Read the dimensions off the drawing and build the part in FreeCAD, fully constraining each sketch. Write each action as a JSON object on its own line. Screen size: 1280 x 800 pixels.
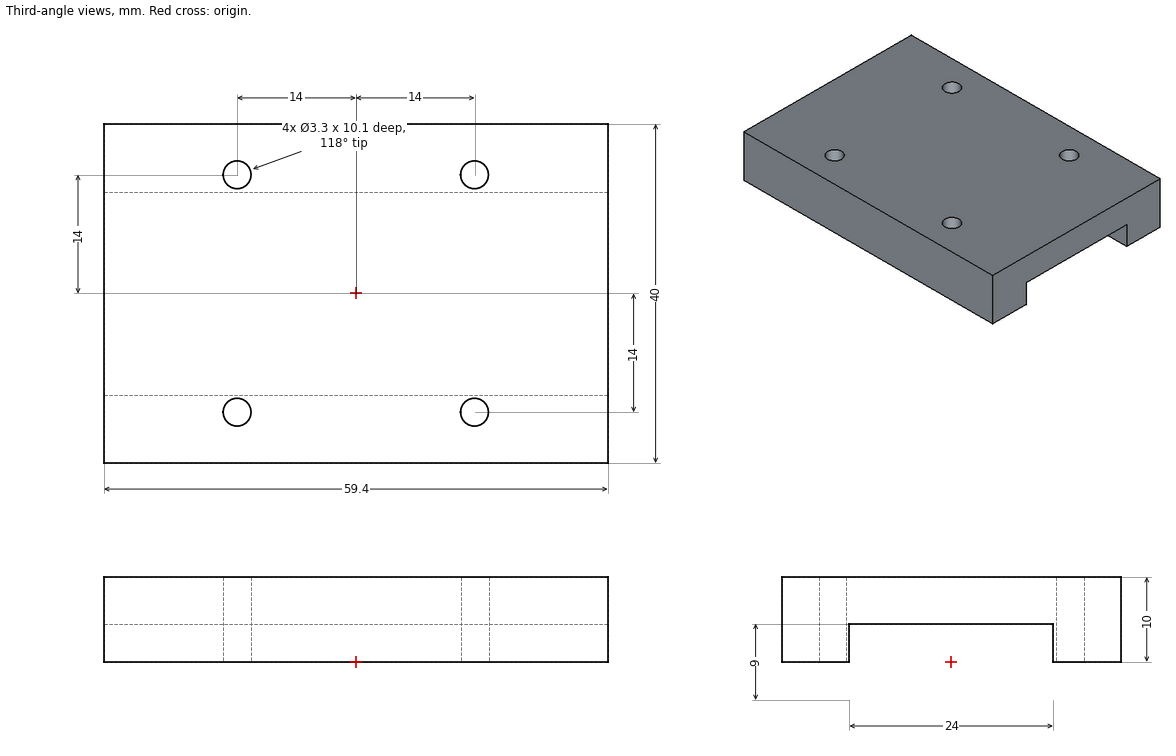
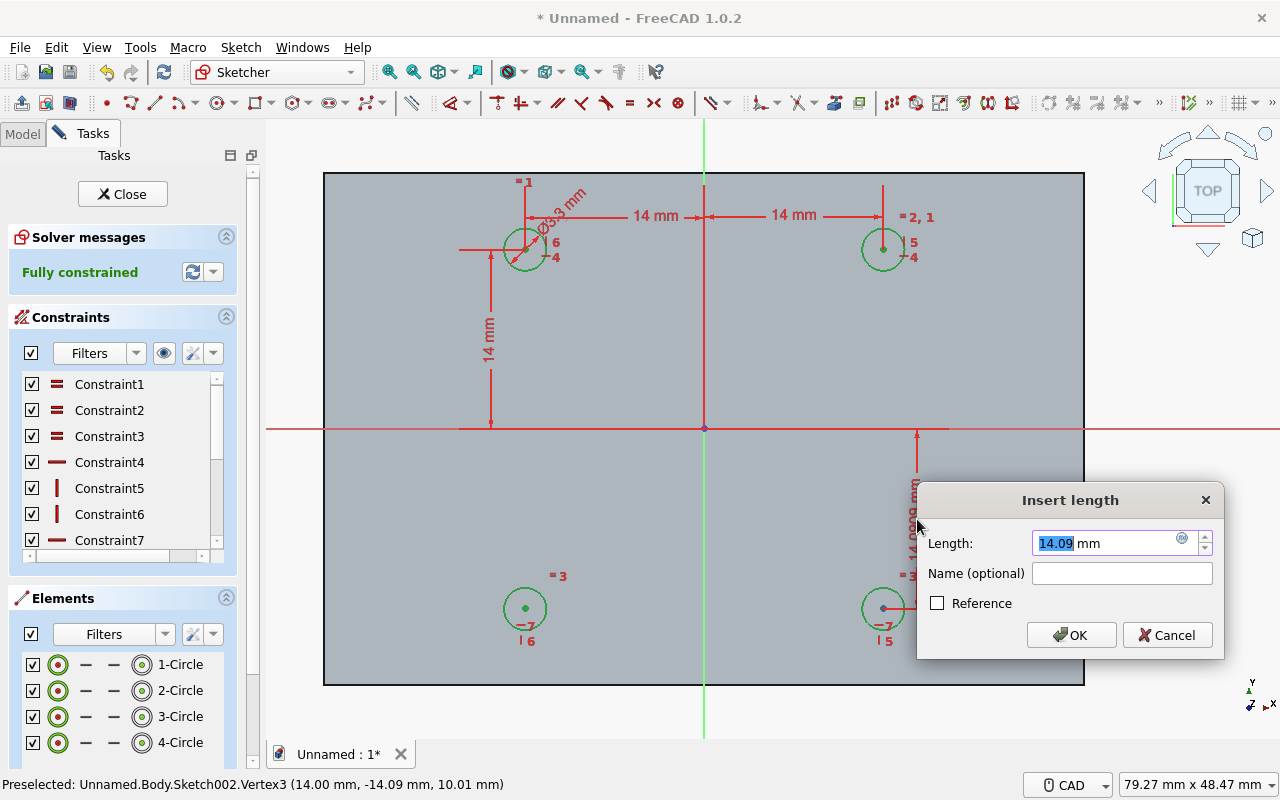
{"action": "type", "text": "14"}
{"action": "key", "text": "Return"}
{"action": "key", "text": "Escape"}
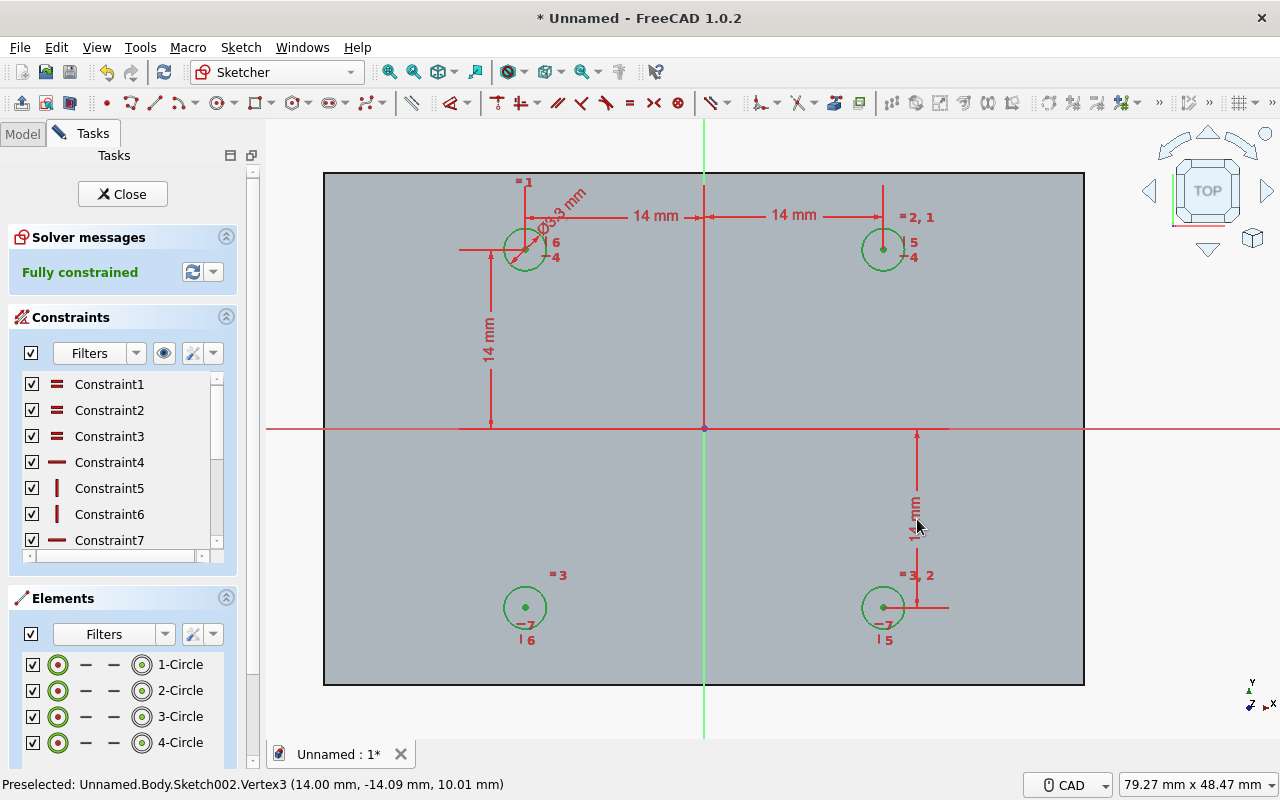
{"action": "left_click", "coordinate": [123, 194]}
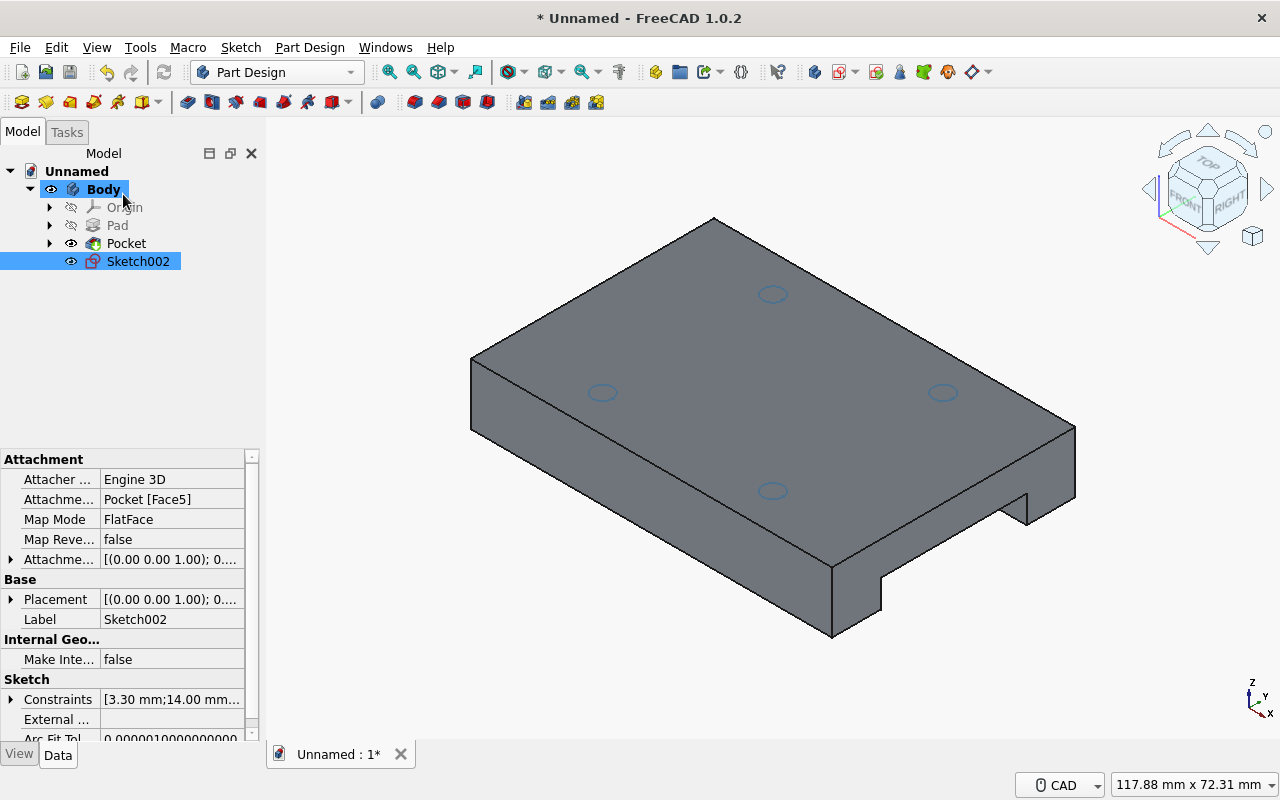
{"action": "left_click", "coordinate": [212, 102]}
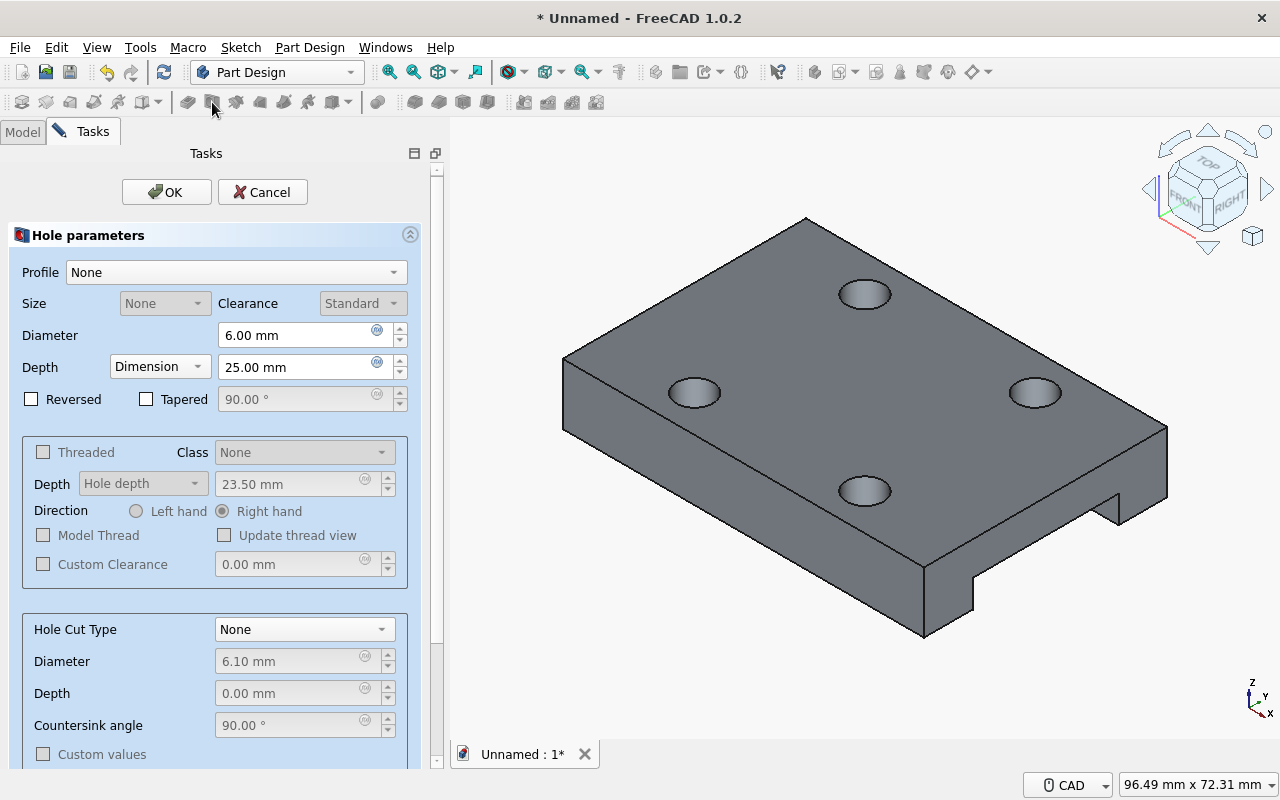
{"action": "triple_click", "coordinate": [305, 335]}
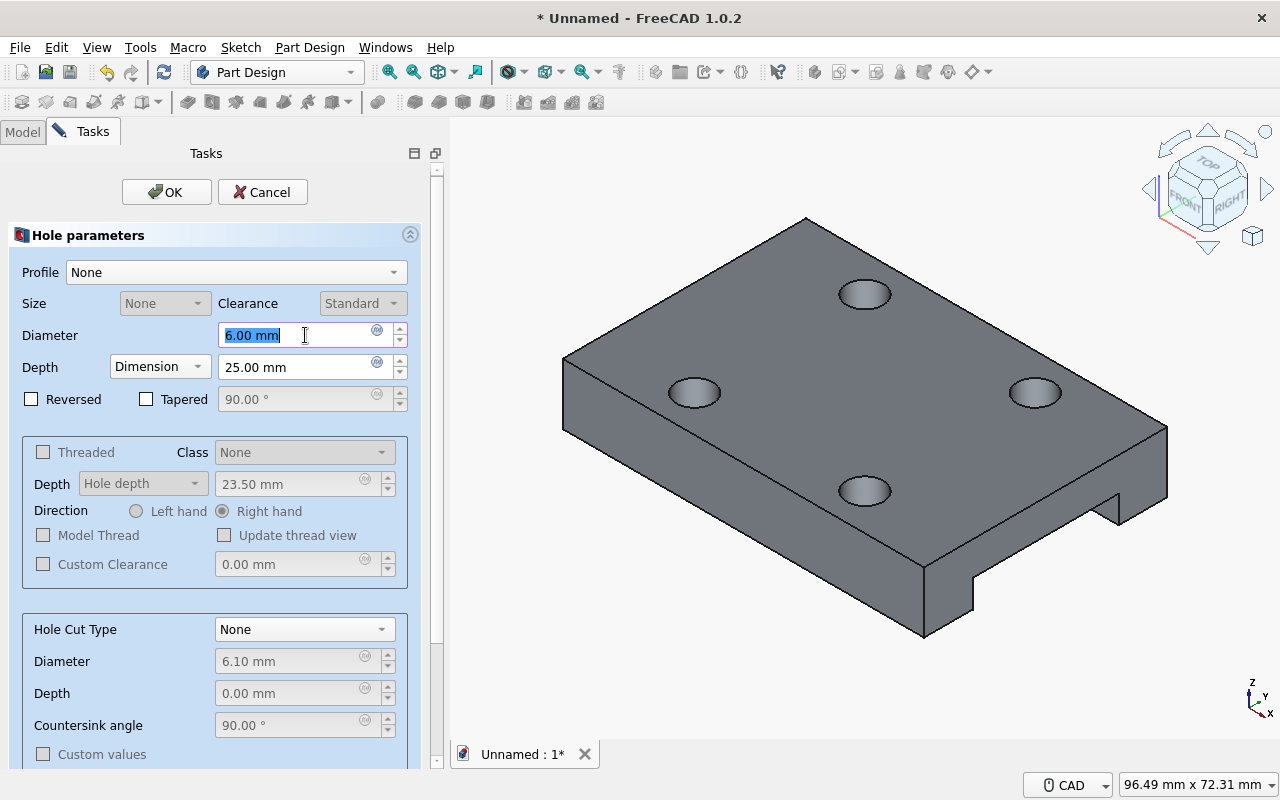
{"action": "type", "text": "3.3"}
{"action": "key", "text": "Tab"}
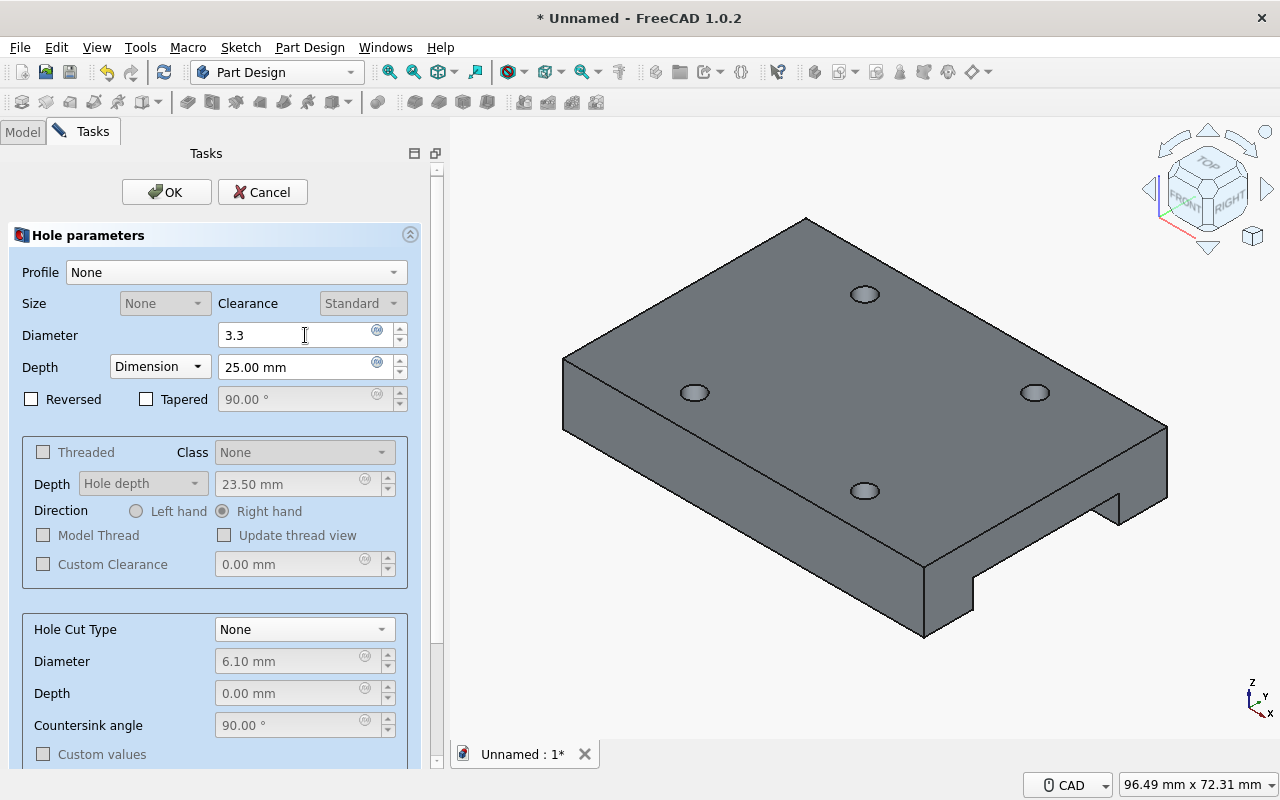
{"action": "triple_click", "coordinate": [305, 367]}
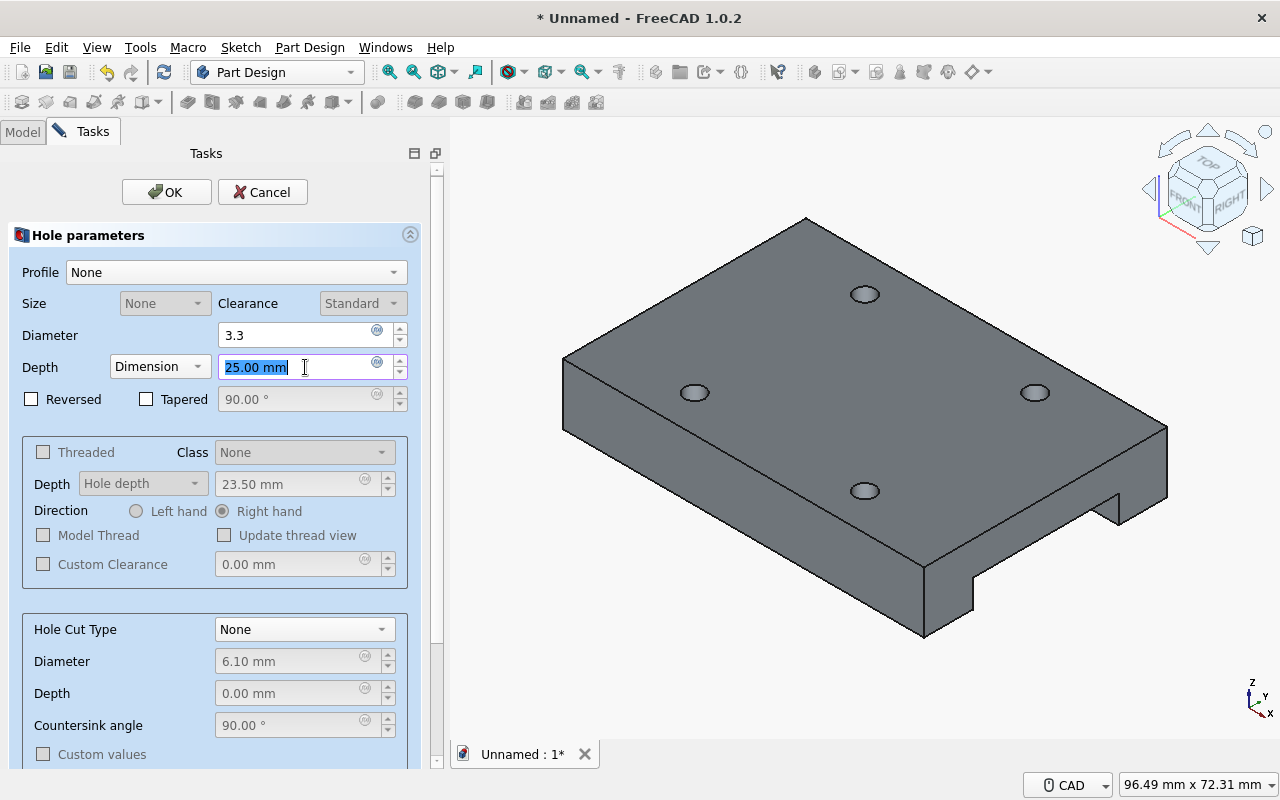
{"action": "type", "text": "10.1"}
{"action": "key", "text": "Tab"}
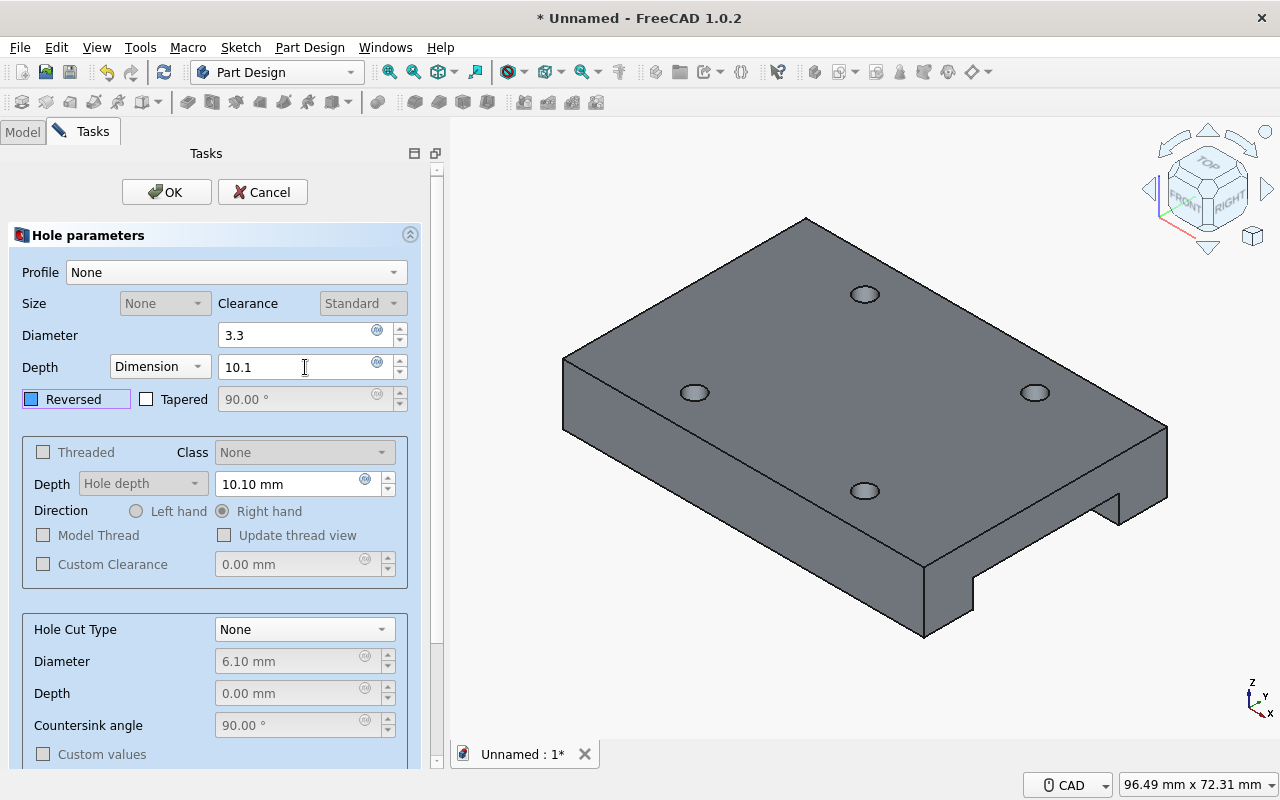
{"action": "left_click", "coordinate": [167, 192]}